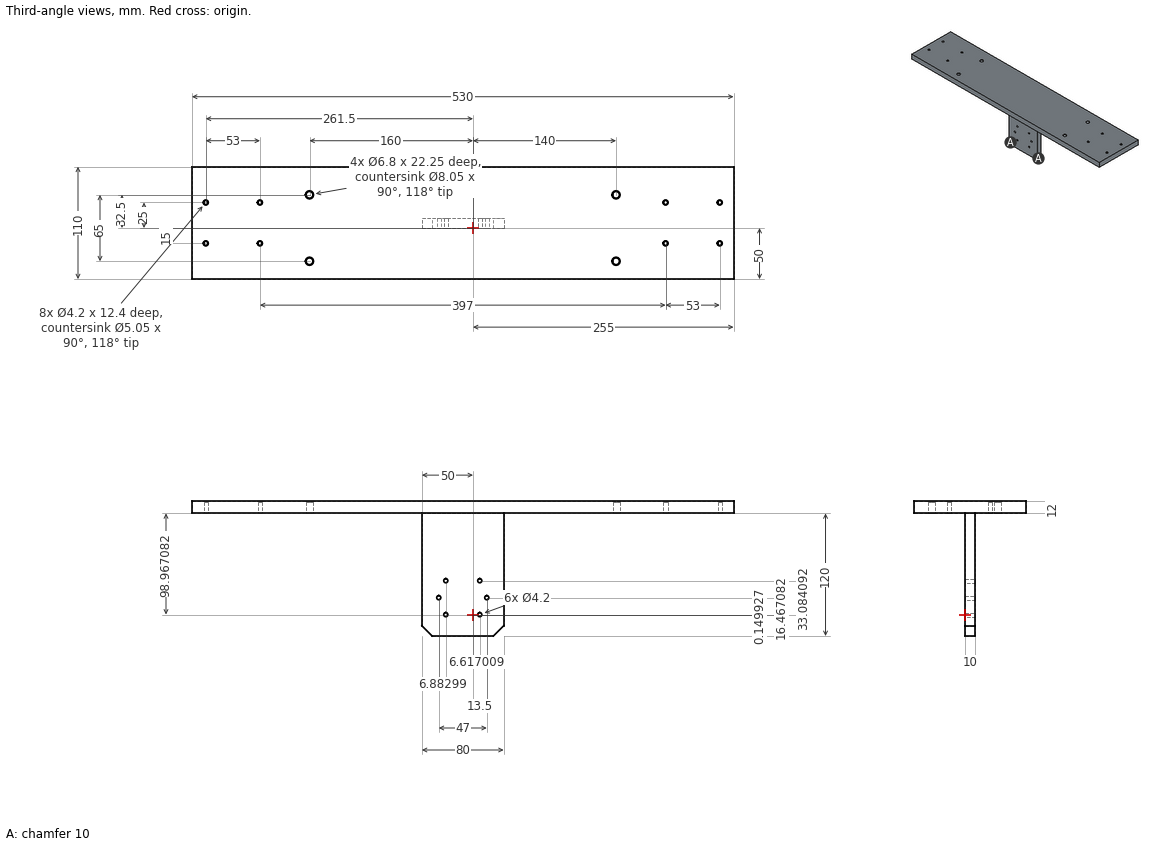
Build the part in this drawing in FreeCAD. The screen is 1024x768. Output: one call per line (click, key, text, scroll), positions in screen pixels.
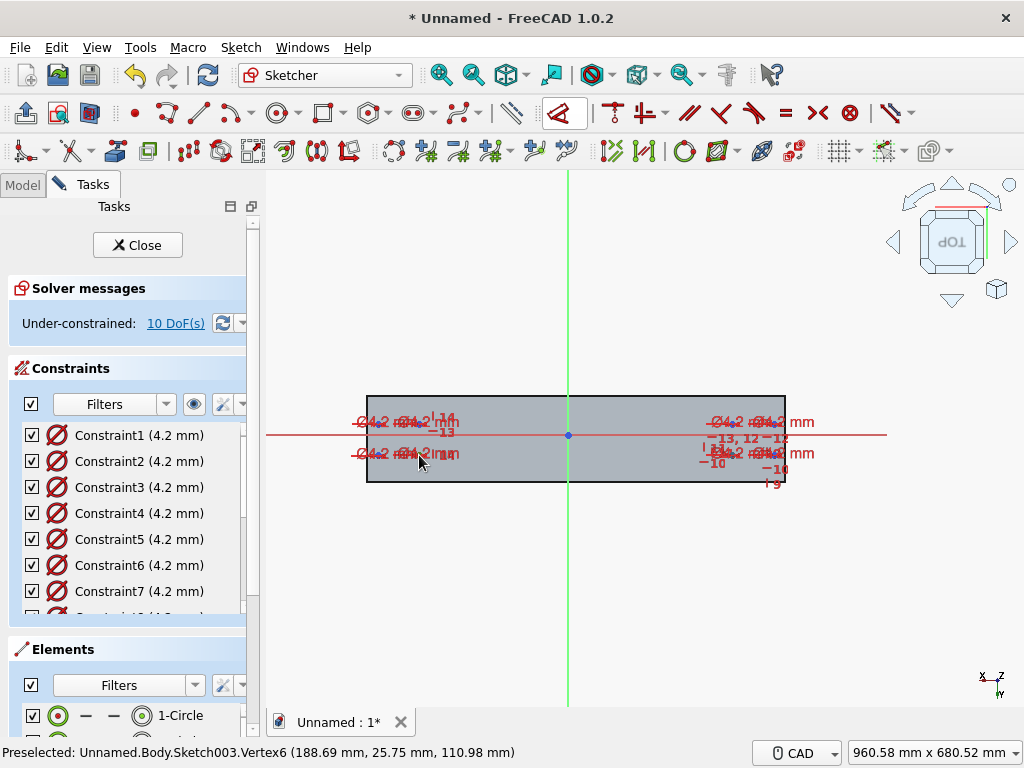
key(h)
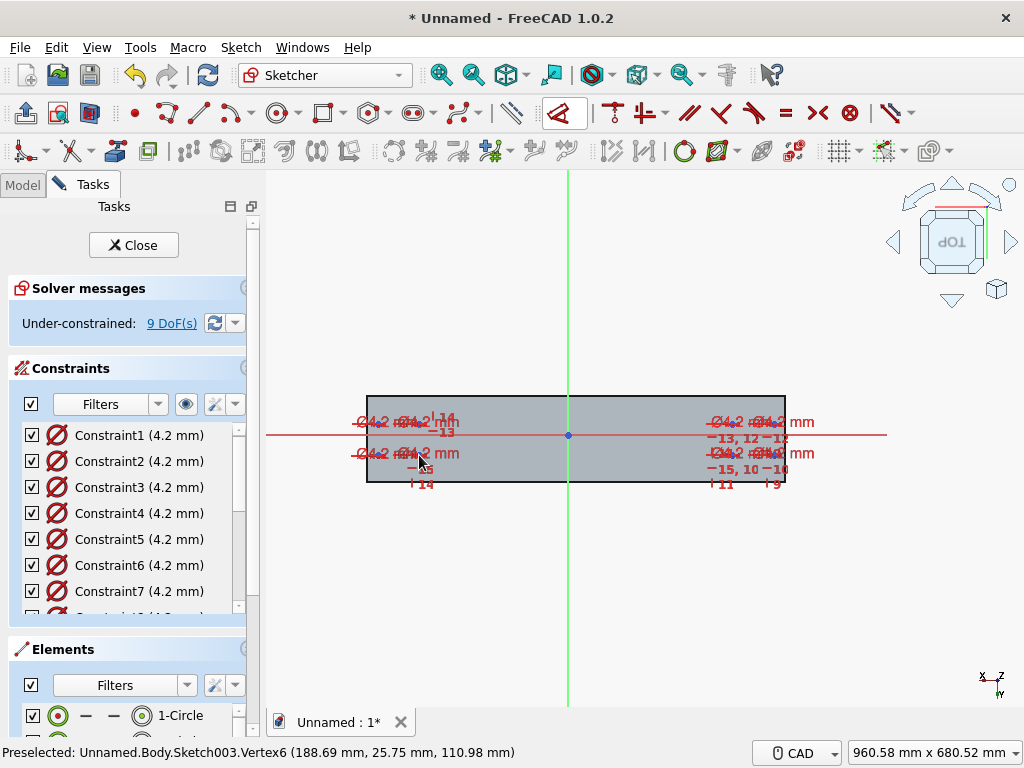
click(419, 424)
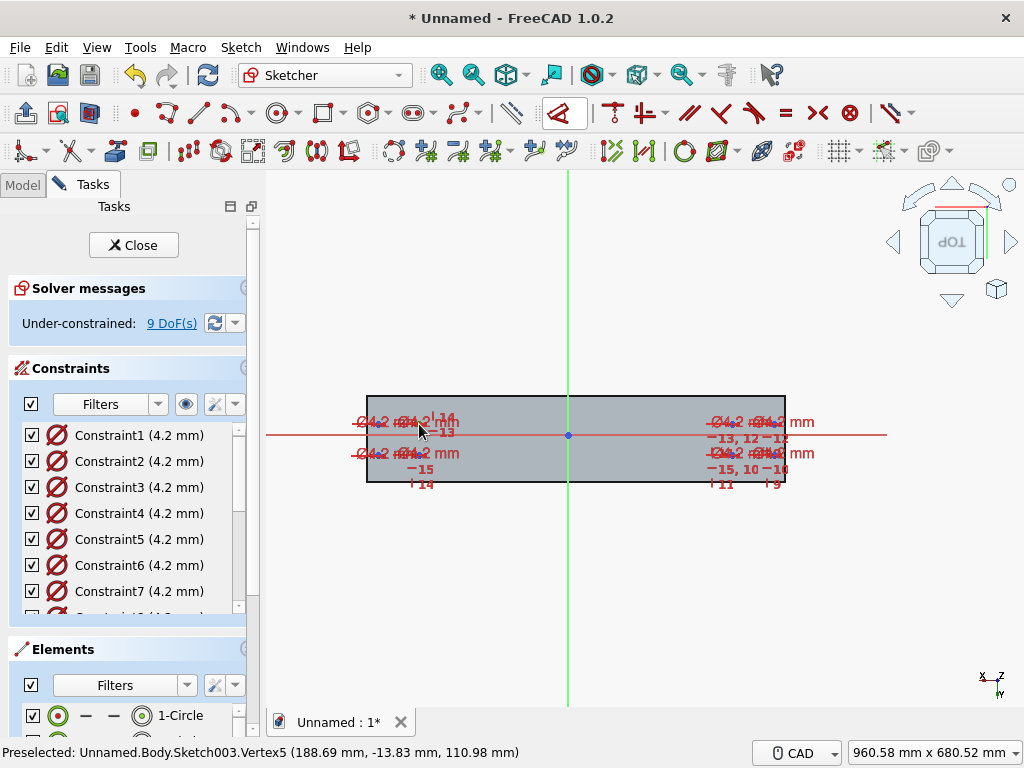
click(378, 424)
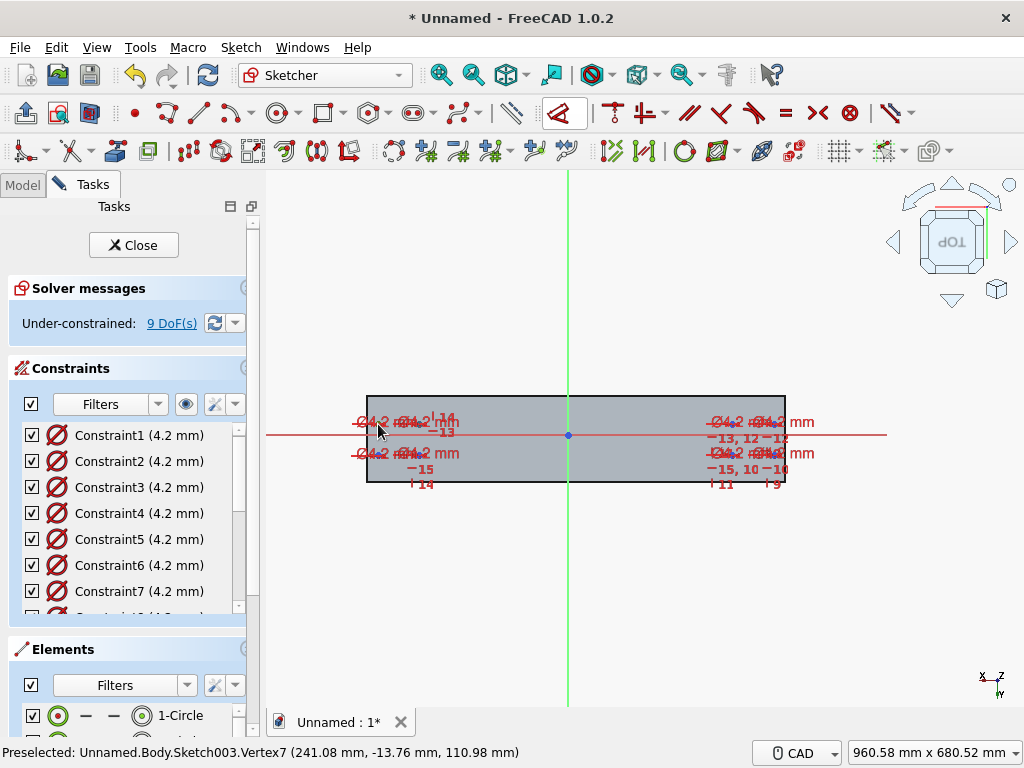
key(h)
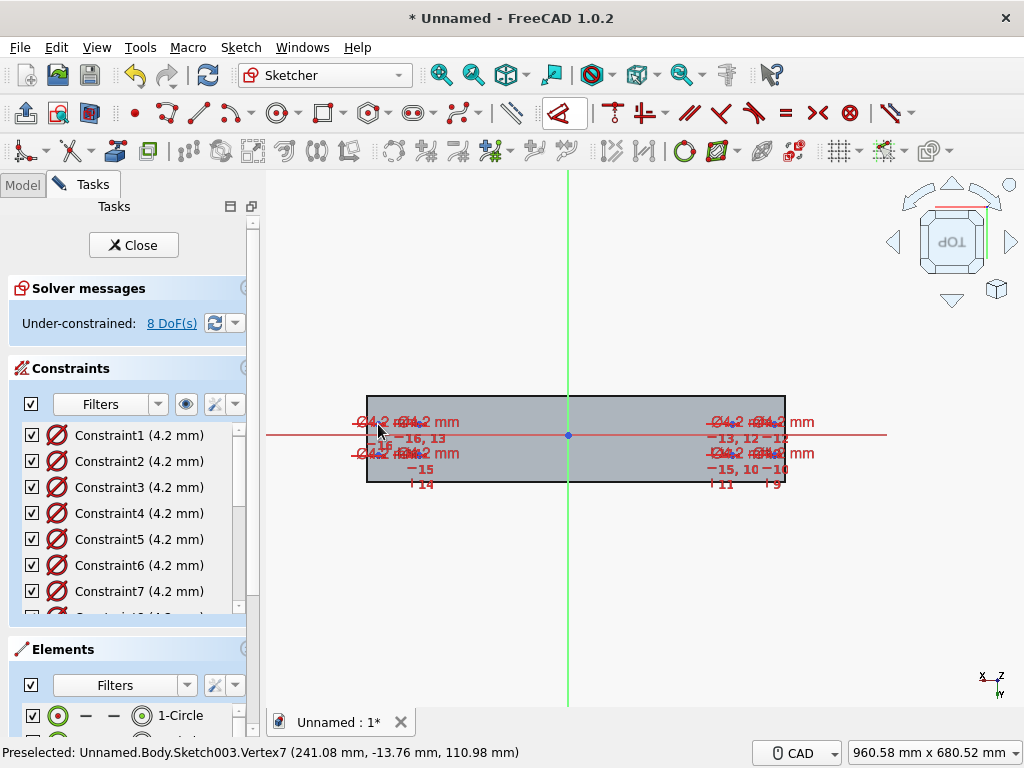
click(378, 424)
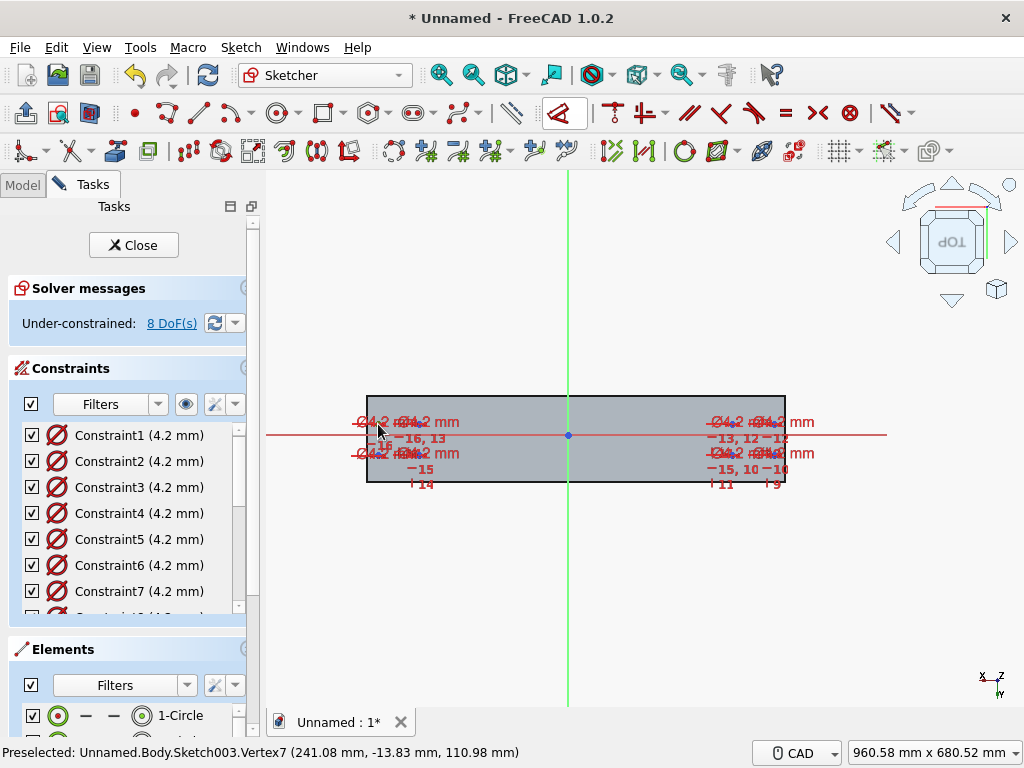
click(378, 456)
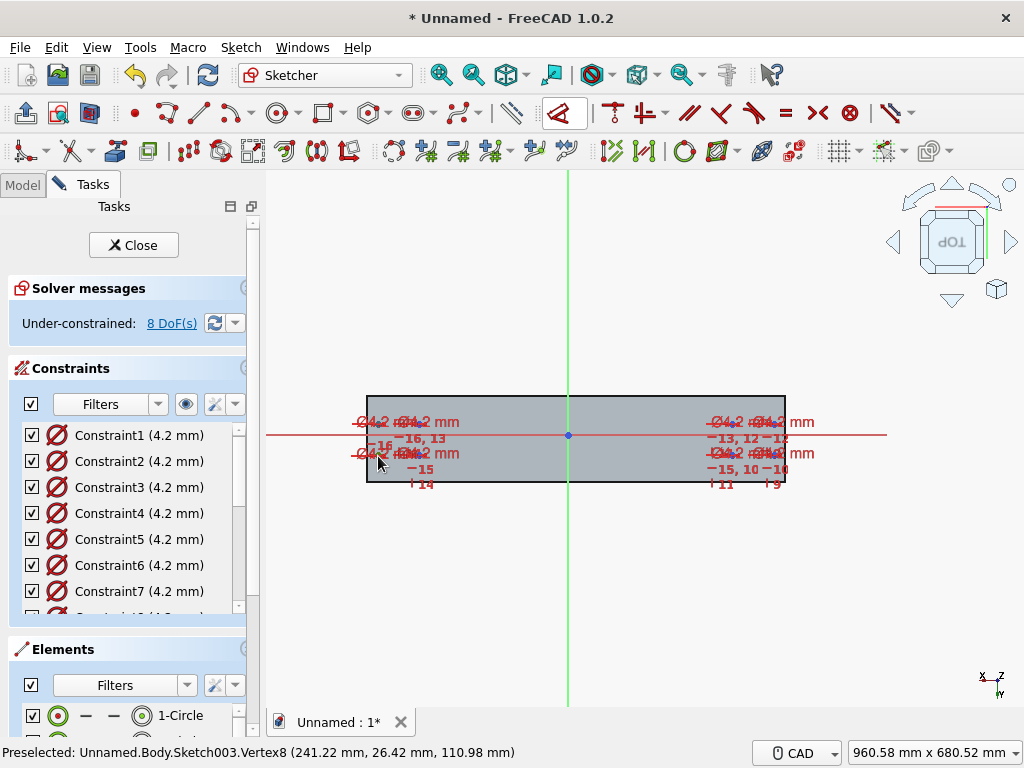
click(668, 114)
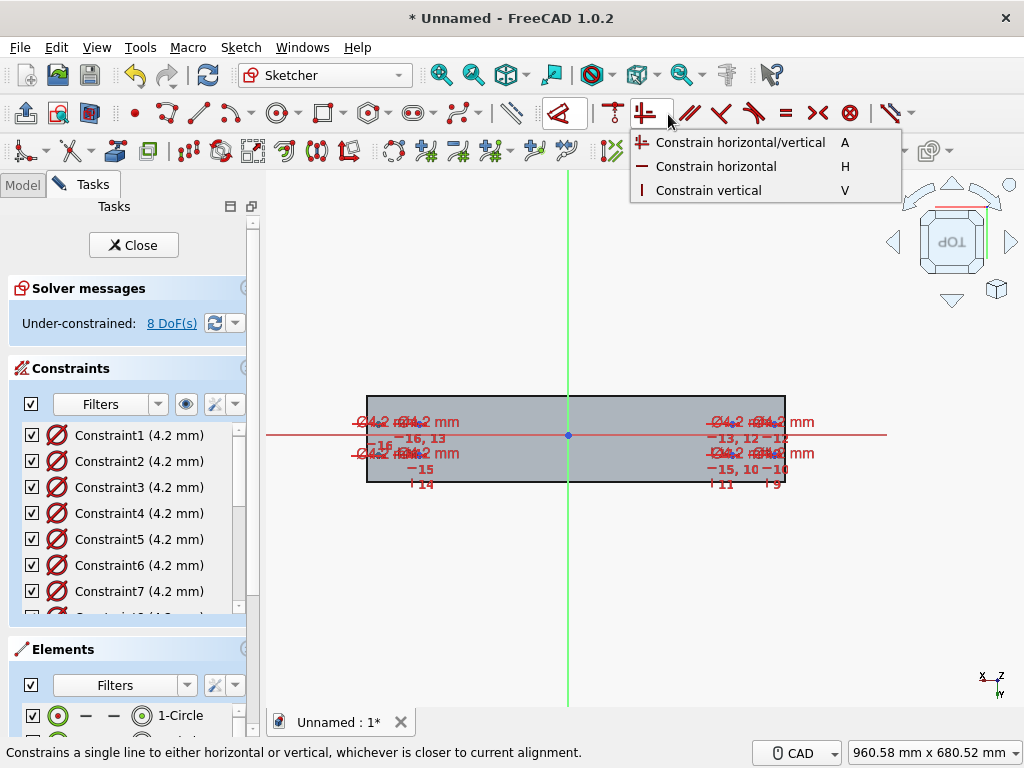
click(766, 190)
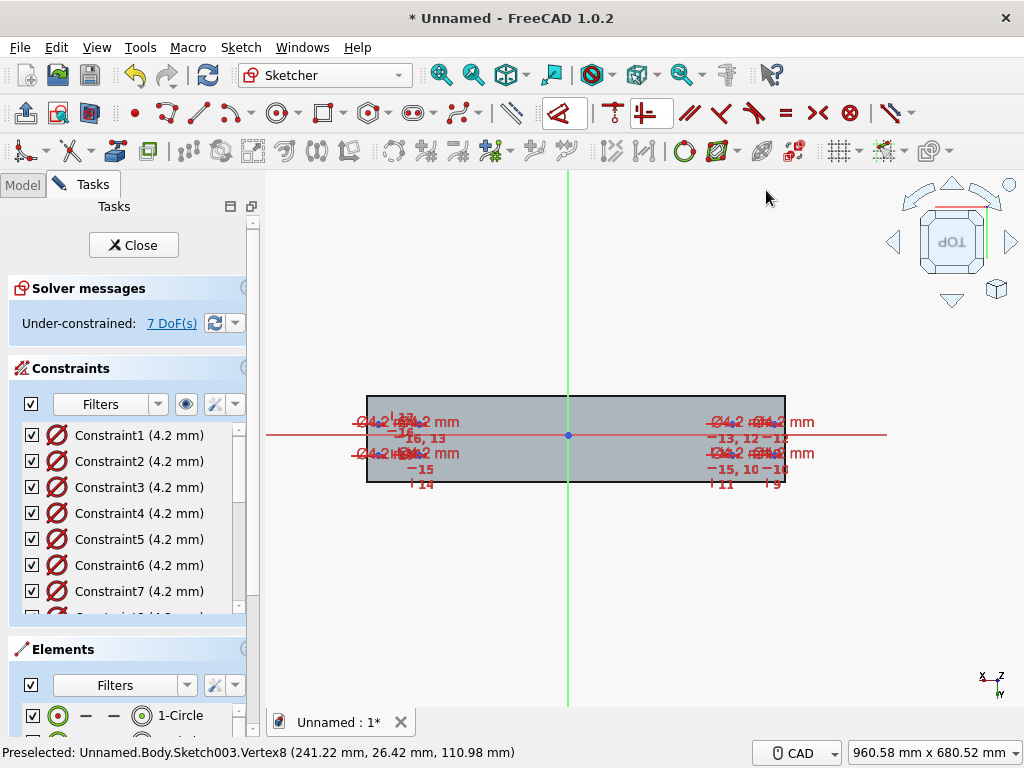
click(419, 455)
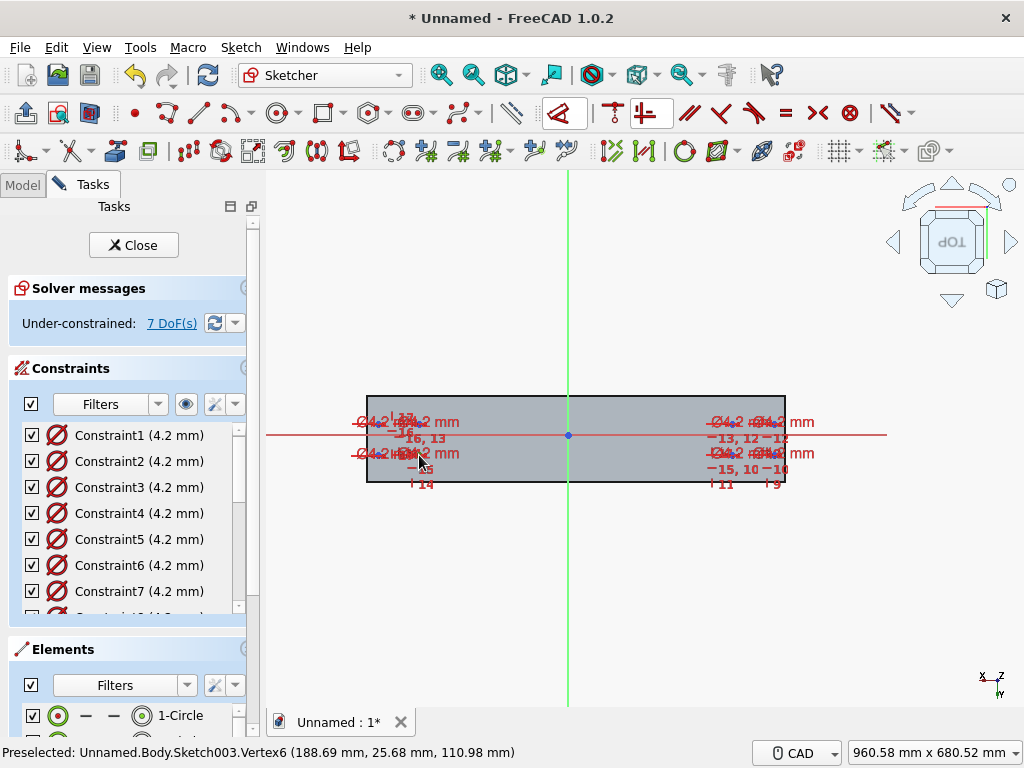
click(378, 456)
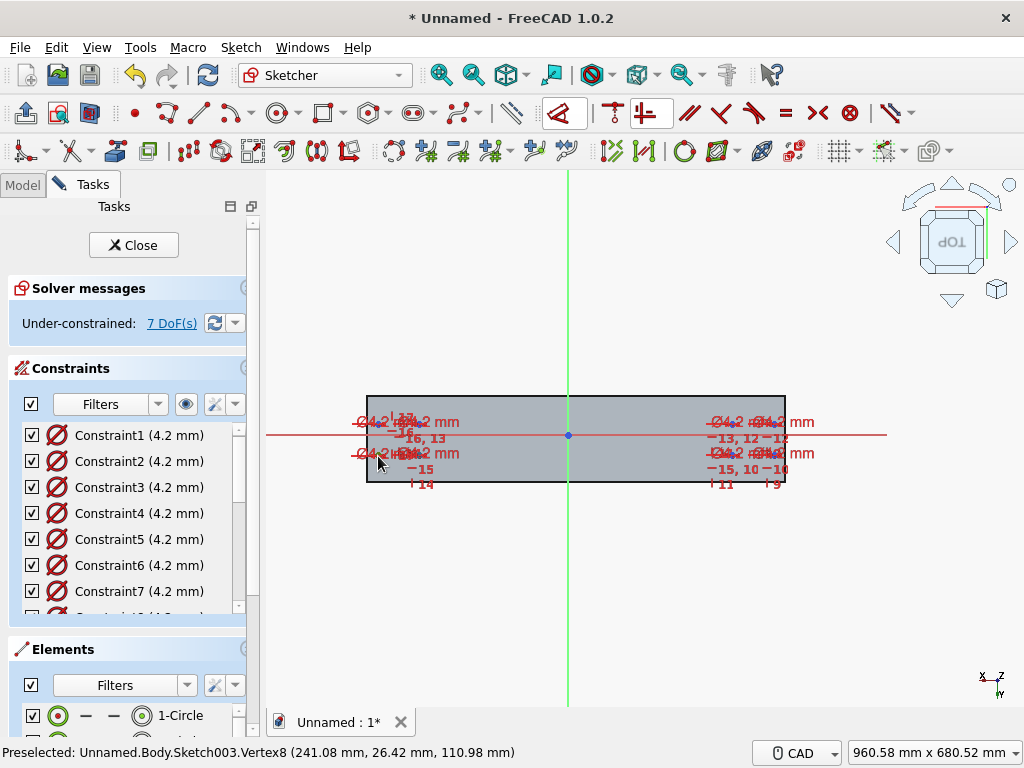
key(h)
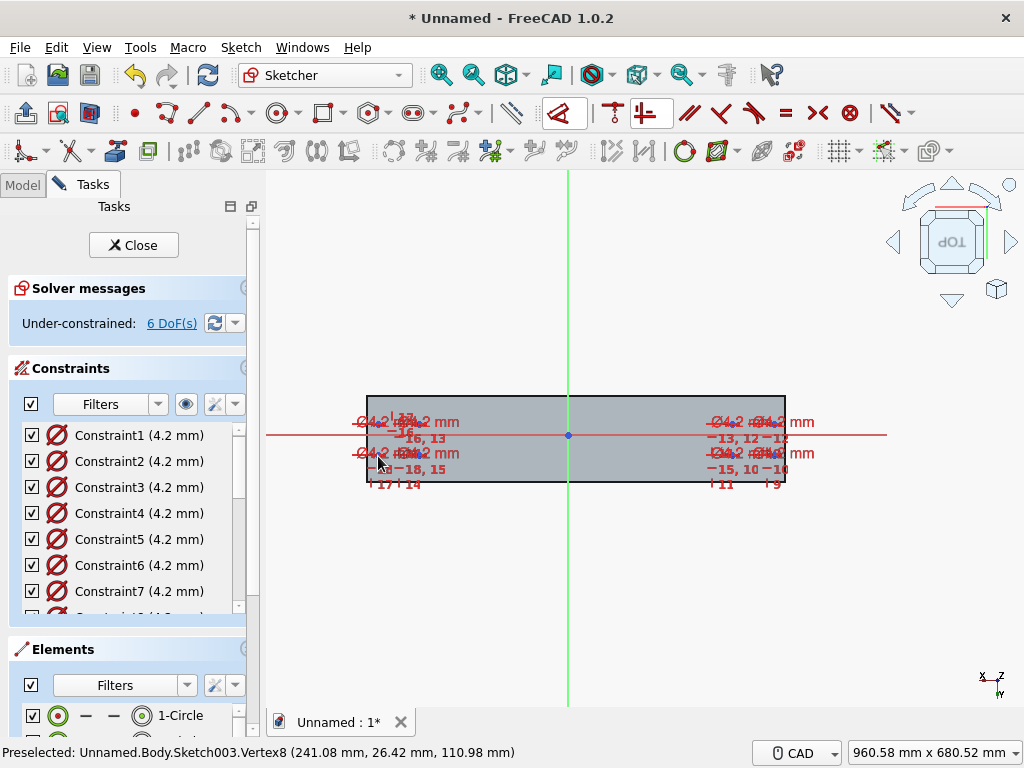
scroll(775, 455, up, 4)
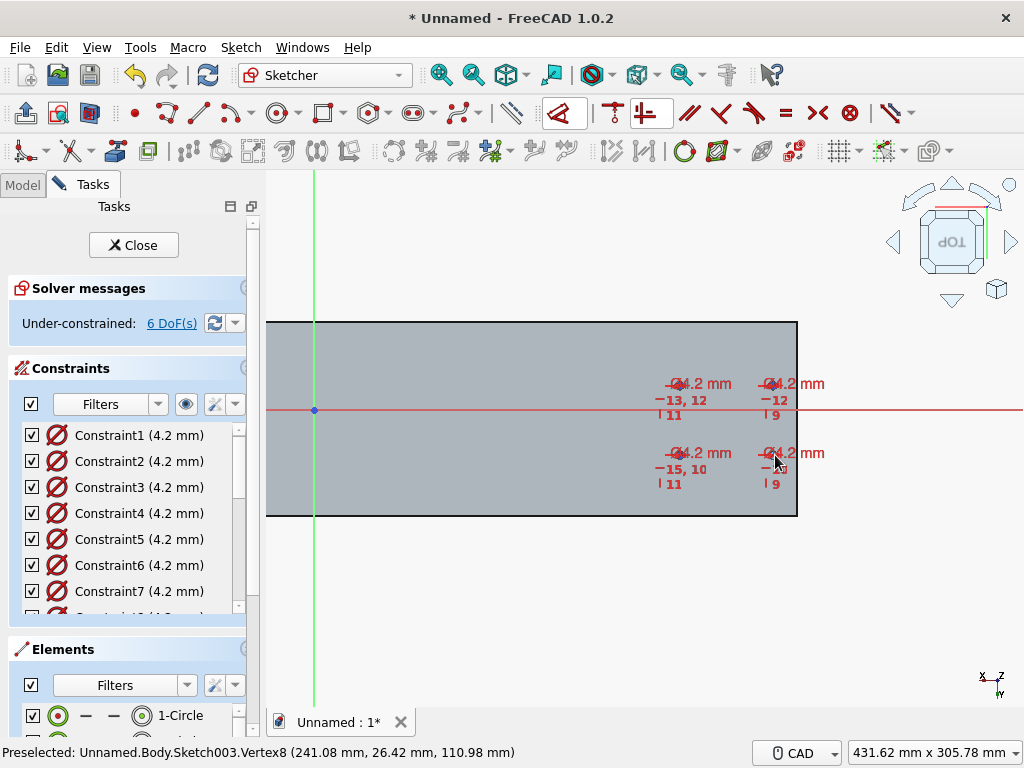
click(773, 455)